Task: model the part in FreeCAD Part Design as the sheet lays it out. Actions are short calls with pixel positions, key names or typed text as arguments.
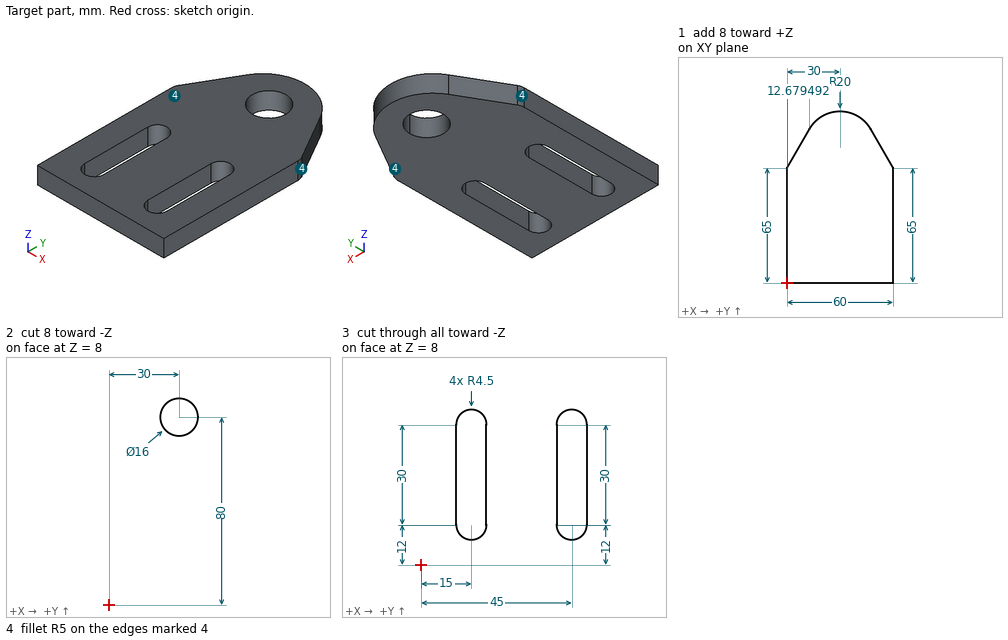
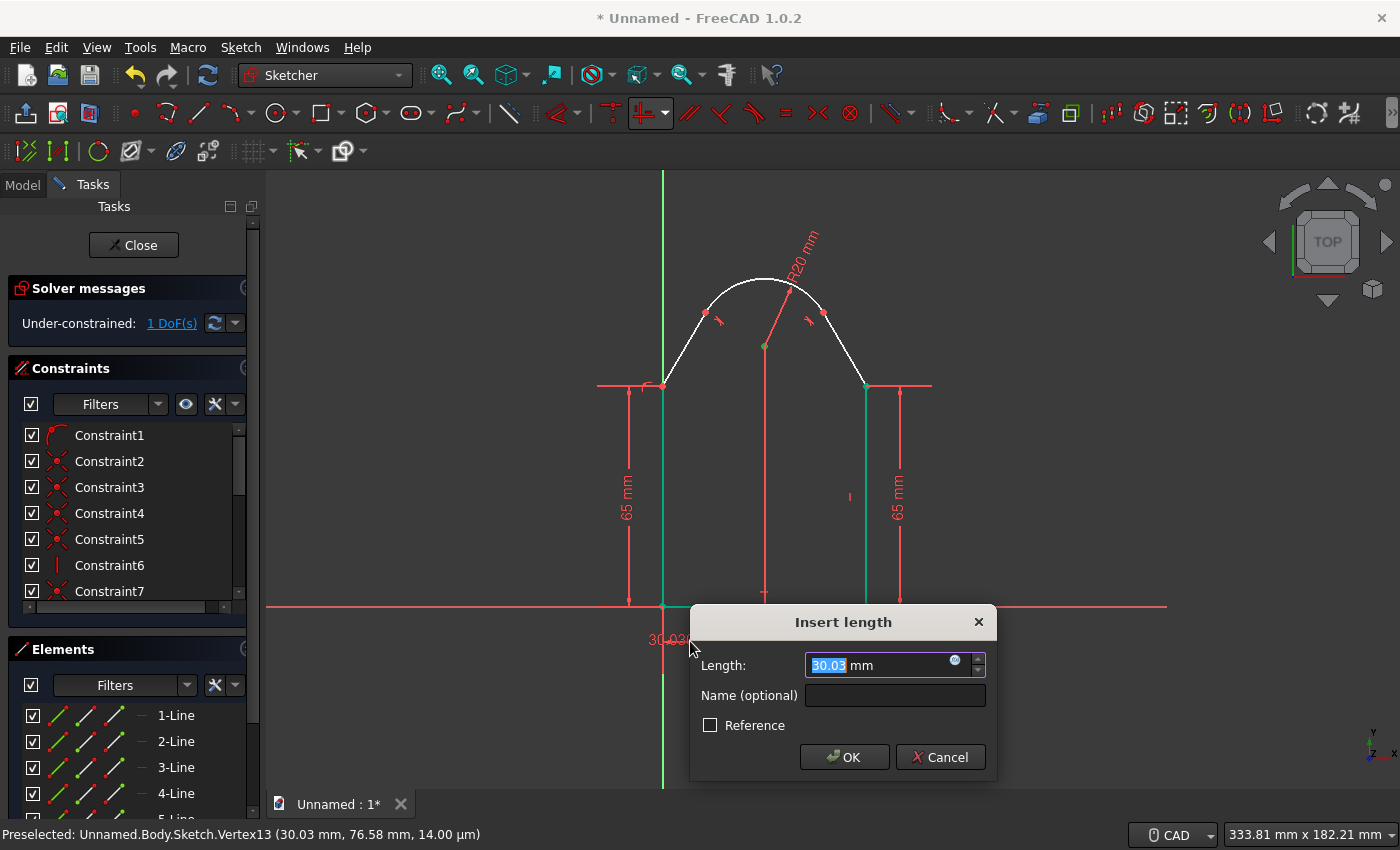
text(30)
key(Return)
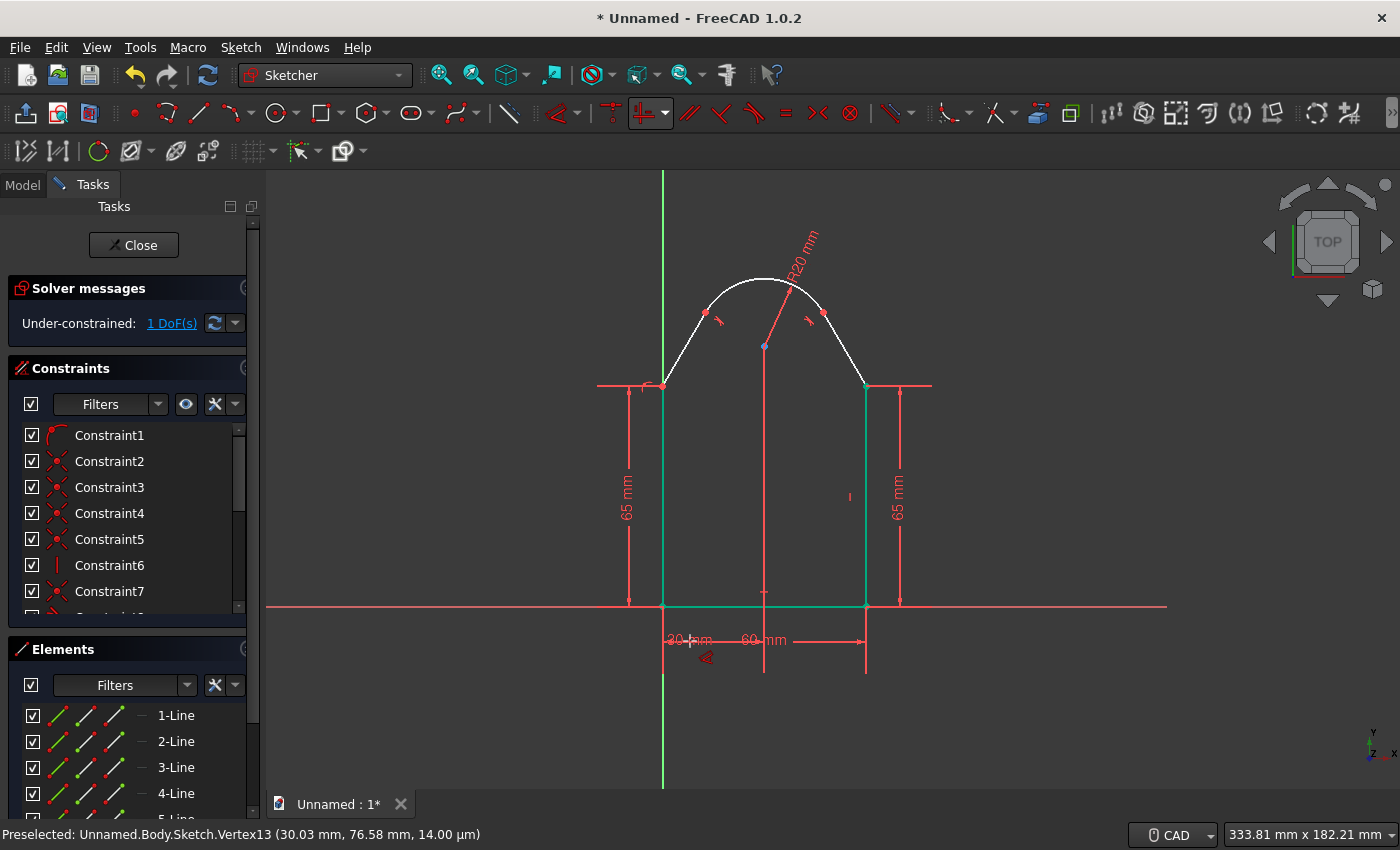
click(706, 312)
click(684, 278)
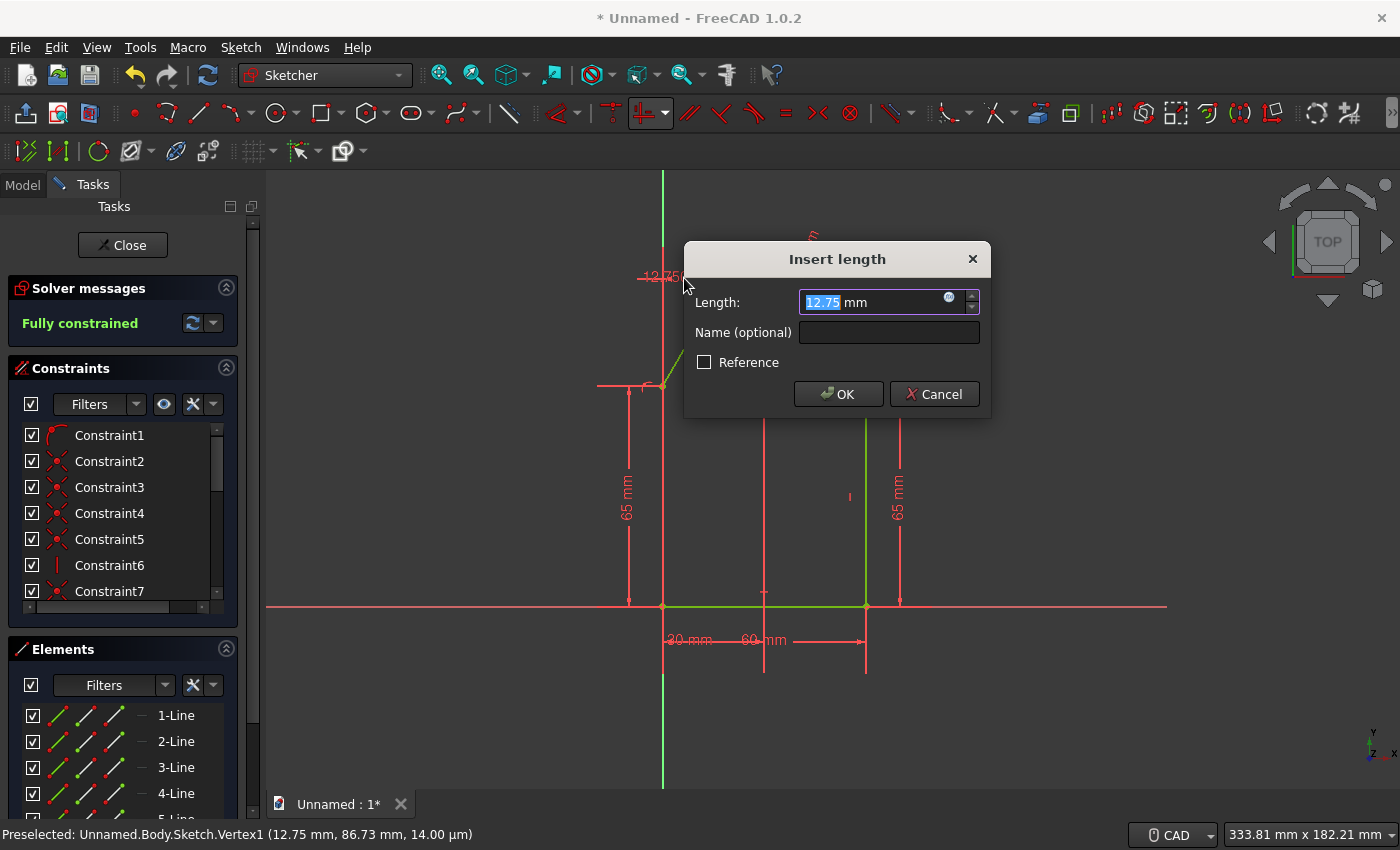
text(12.679492)
key(Return)
key(Escape)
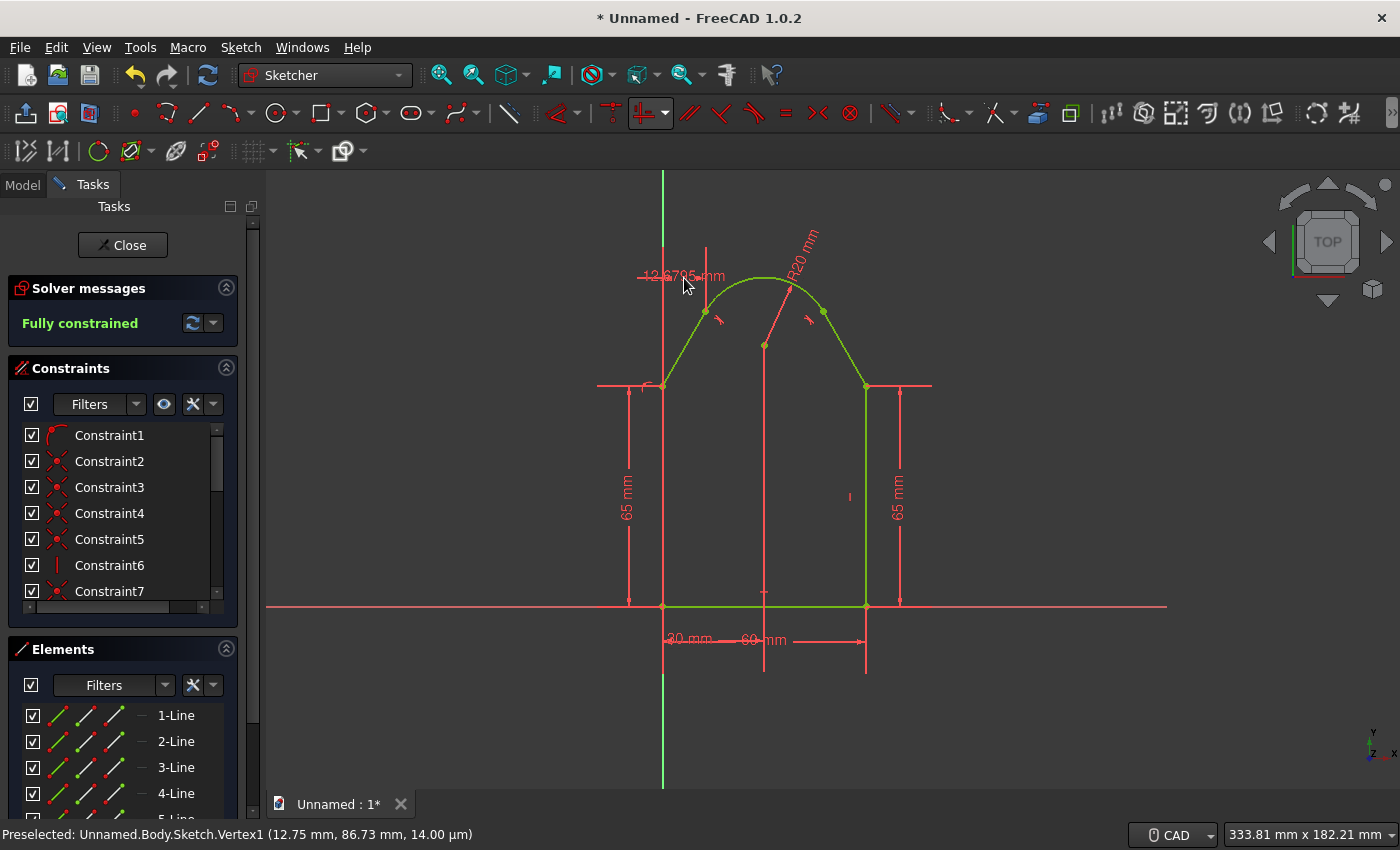
click(123, 245)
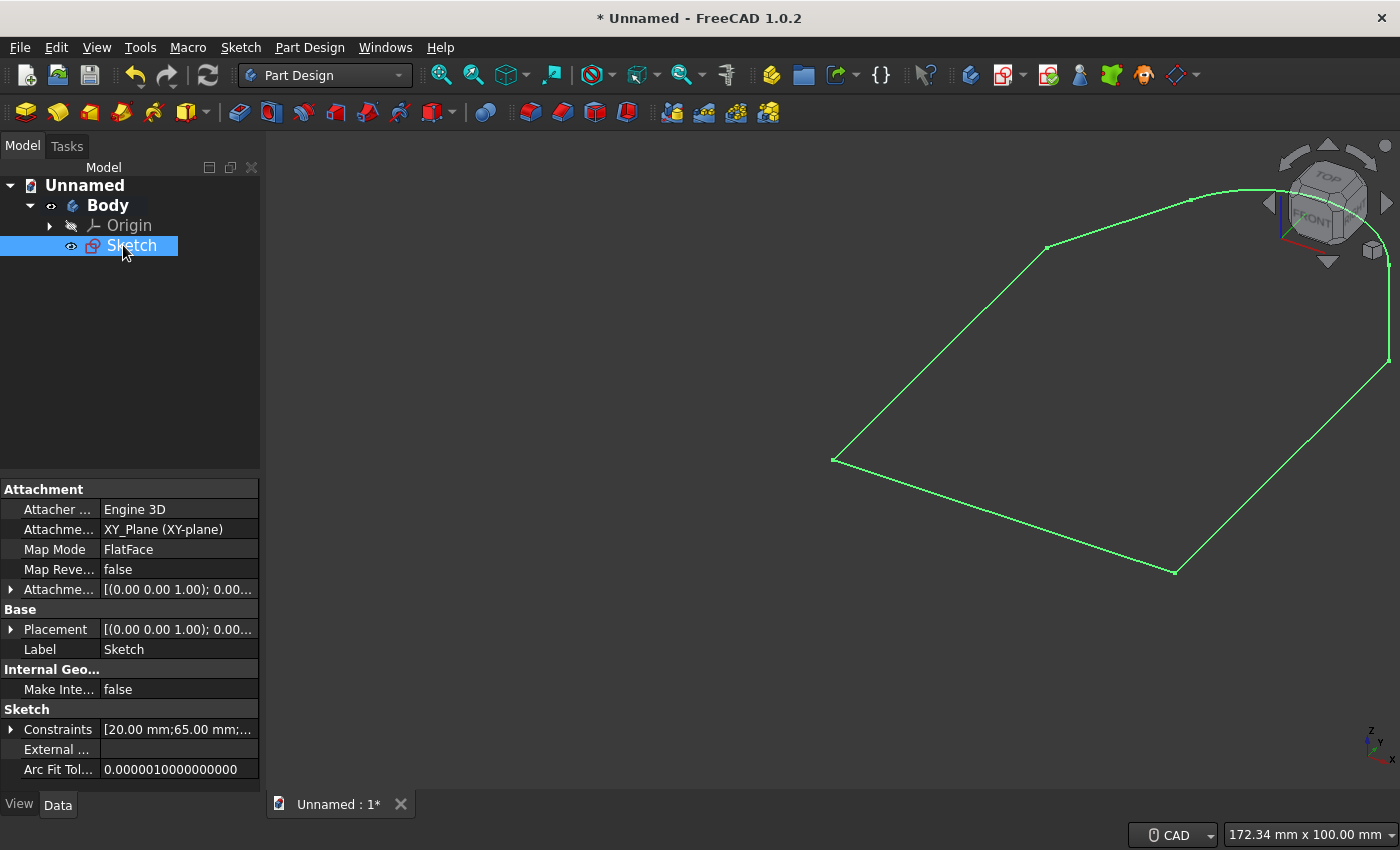
click(26, 112)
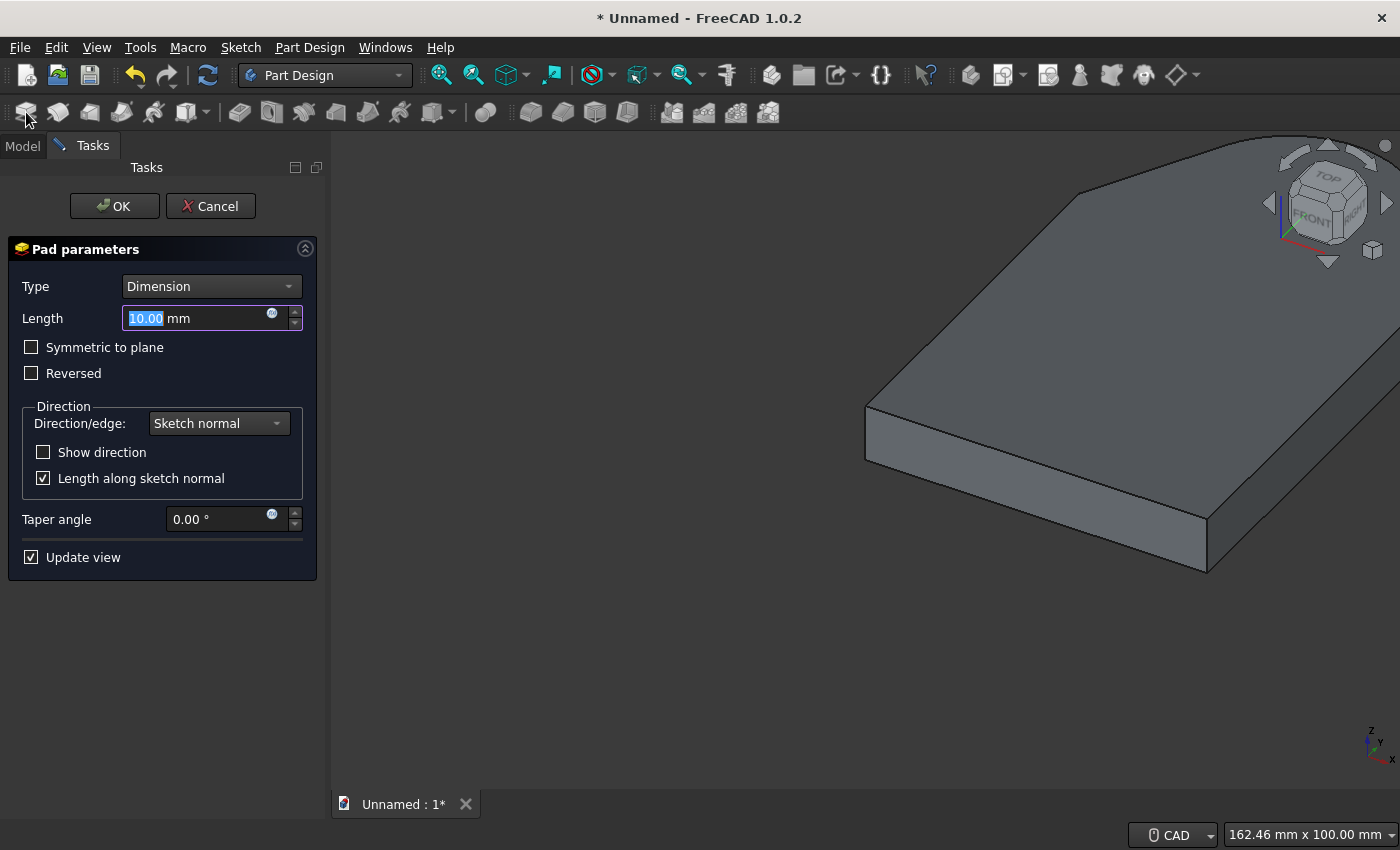
text(8)
key(Tab)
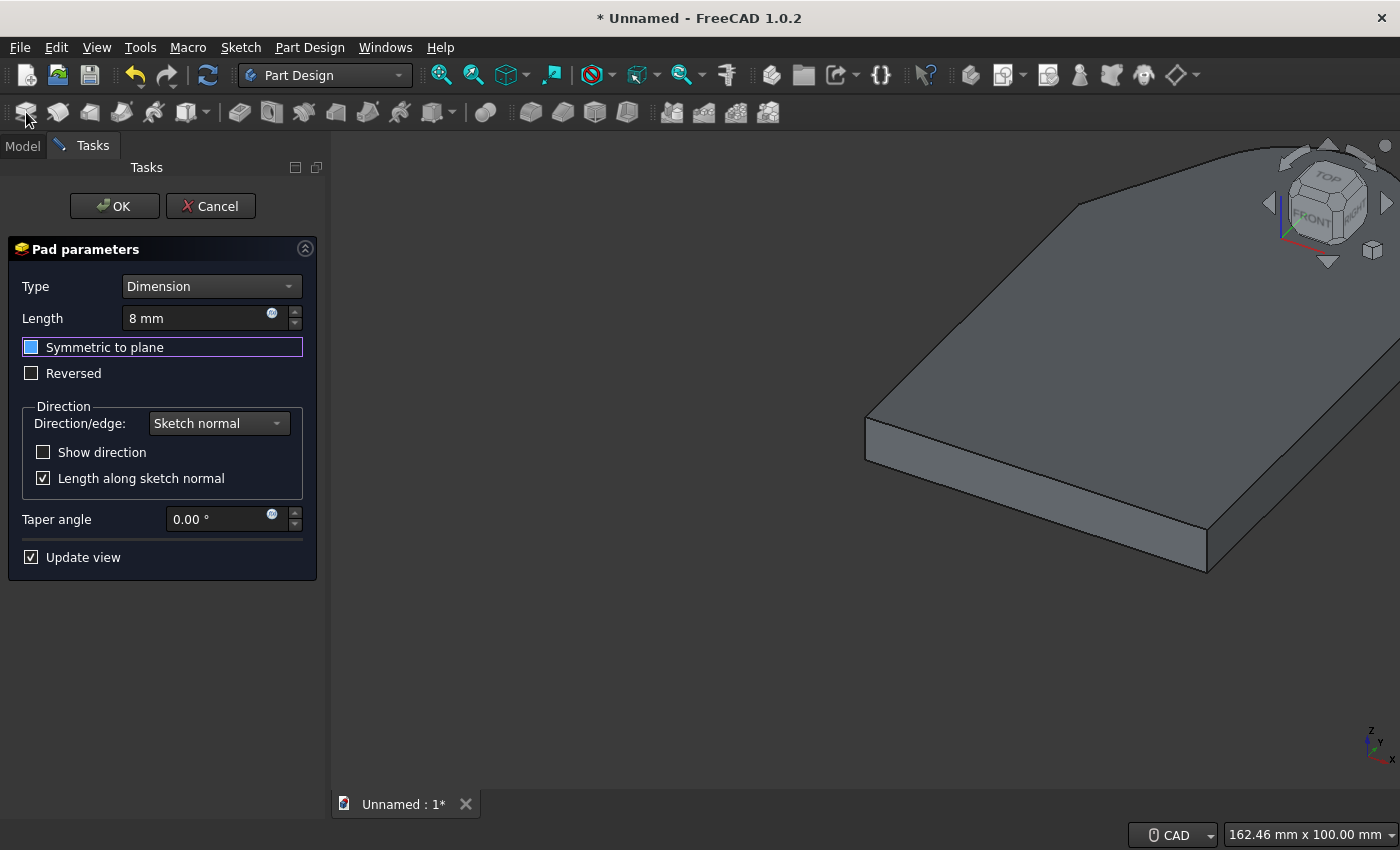
click(115, 206)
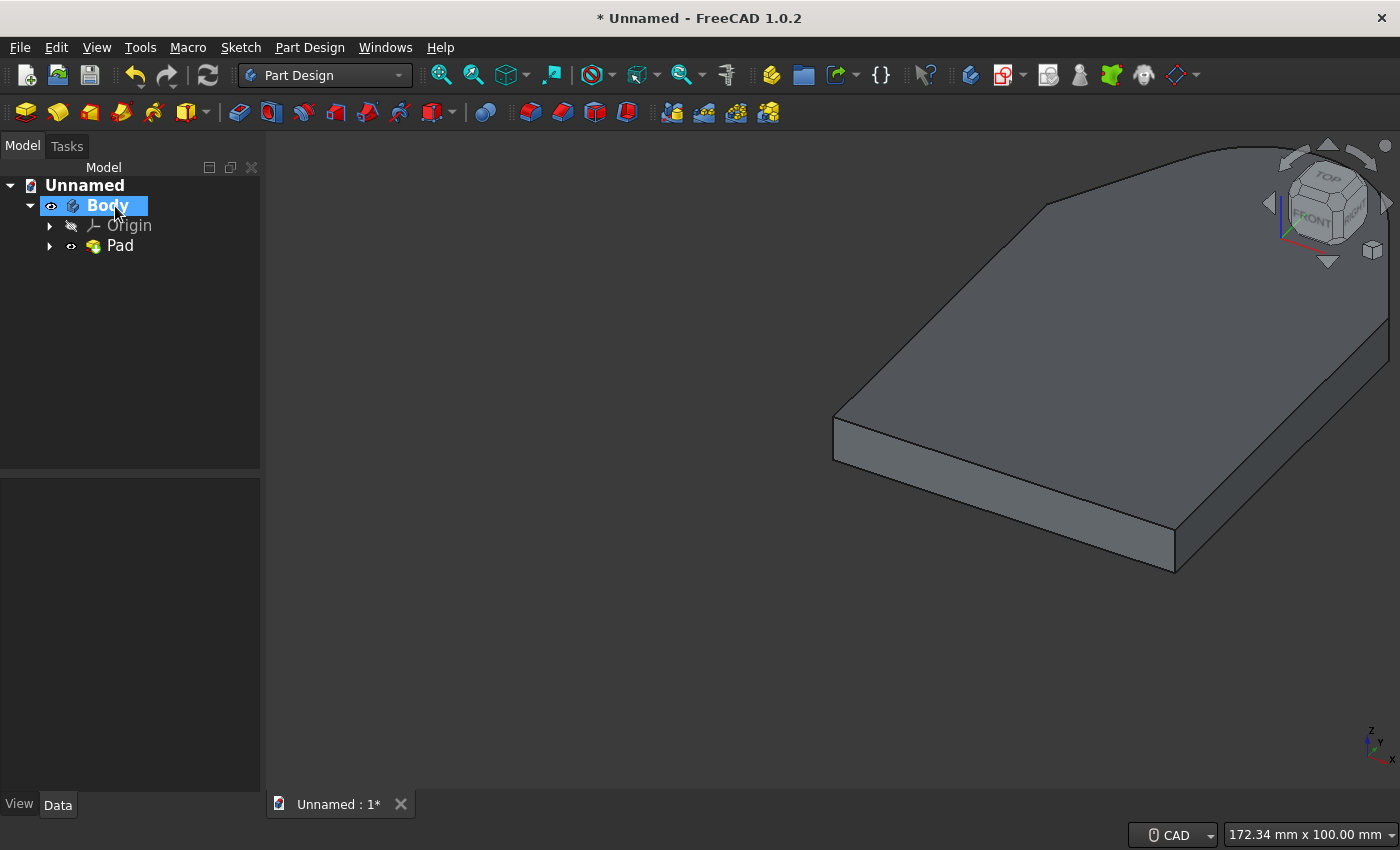
key(v)
key(f)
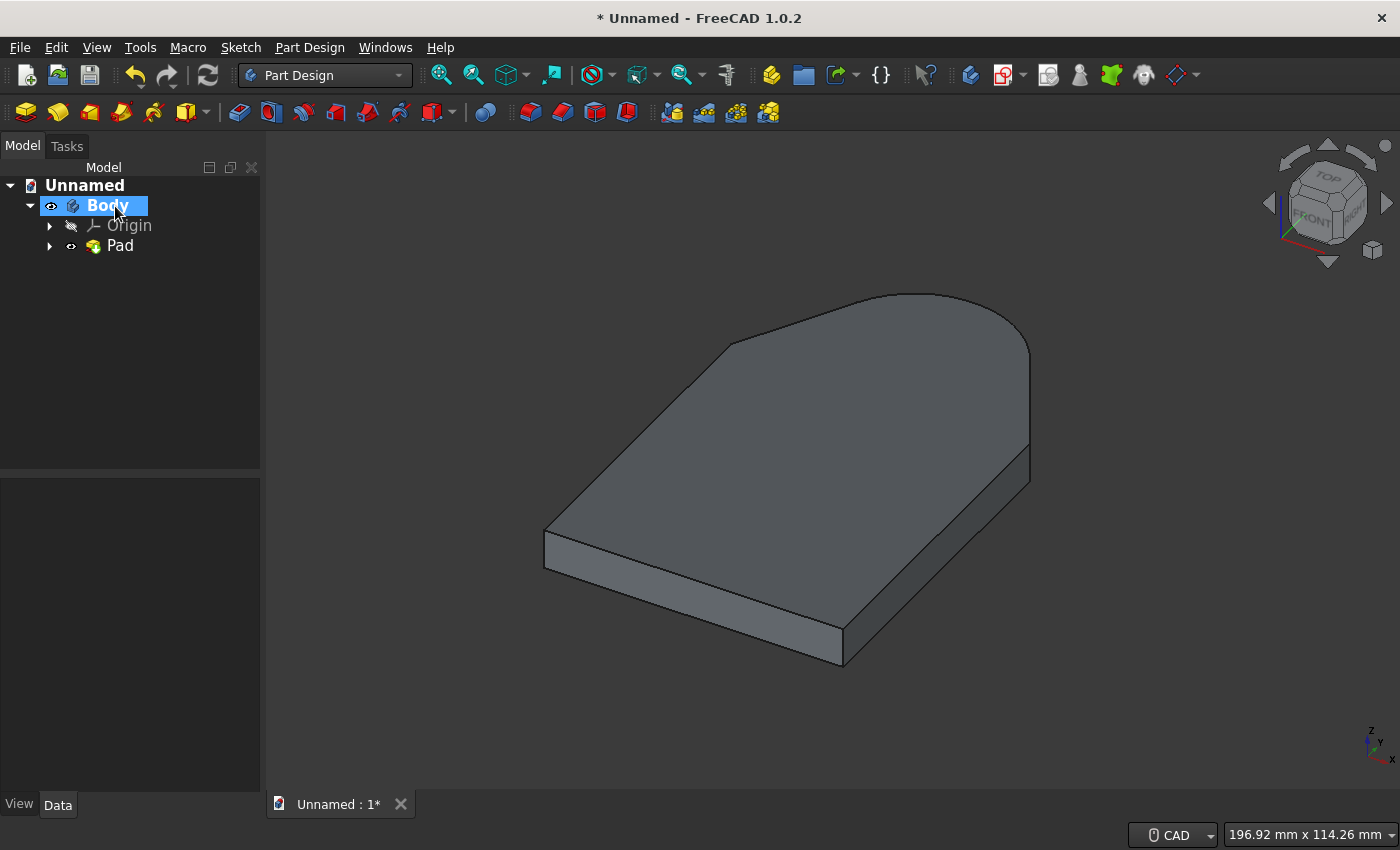
click(833, 440)